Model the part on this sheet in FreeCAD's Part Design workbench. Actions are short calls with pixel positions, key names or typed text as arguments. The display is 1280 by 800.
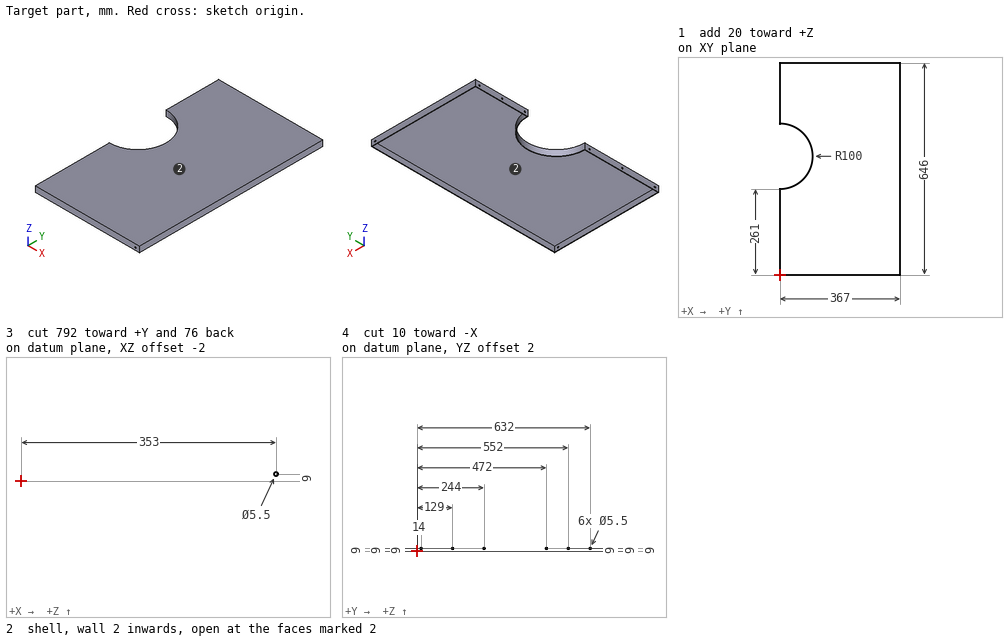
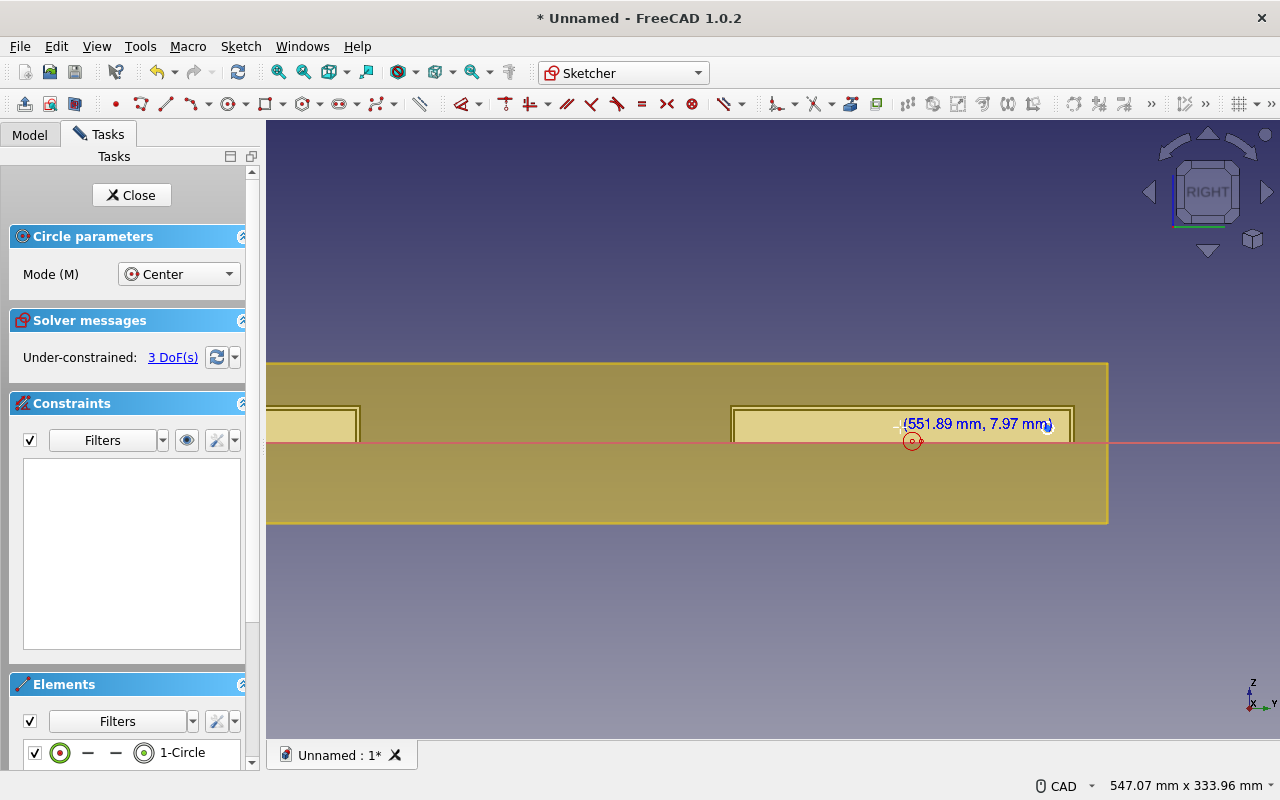
click(899, 427)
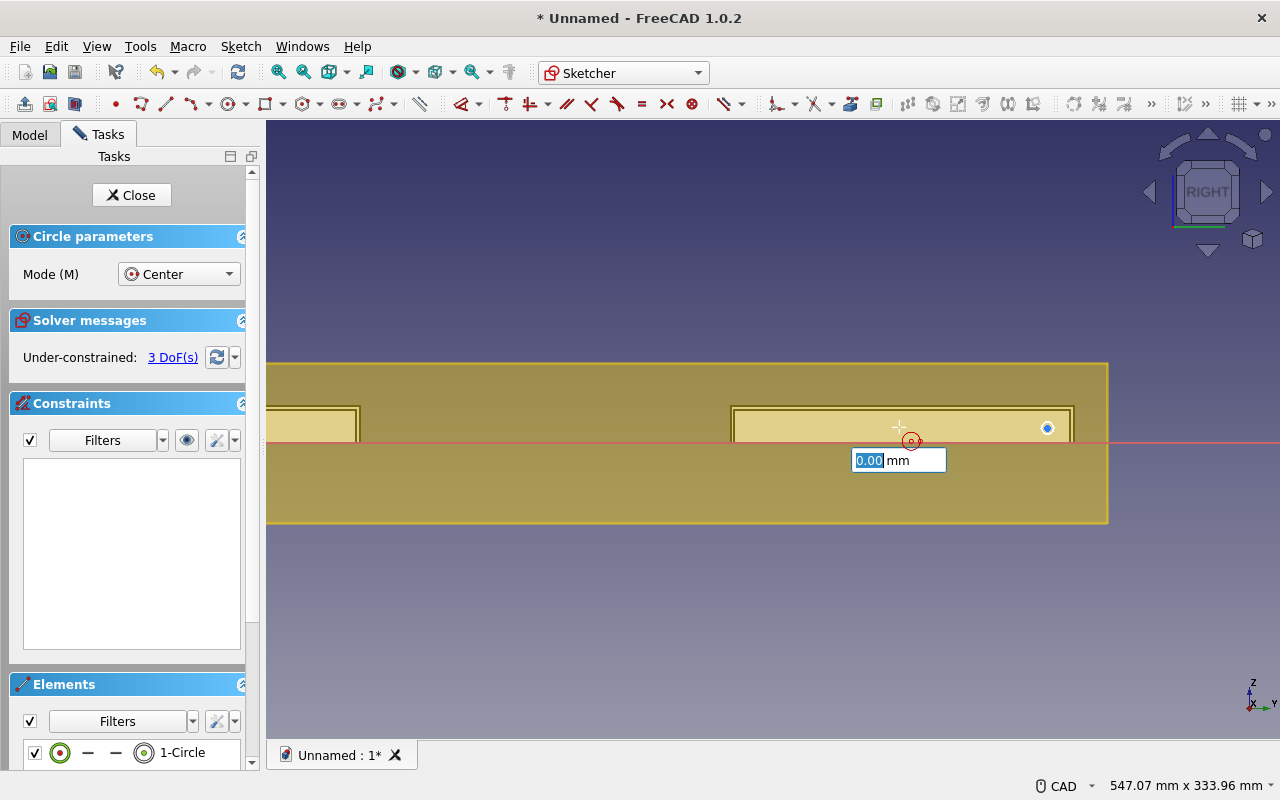
scroll(903, 423, up, 6)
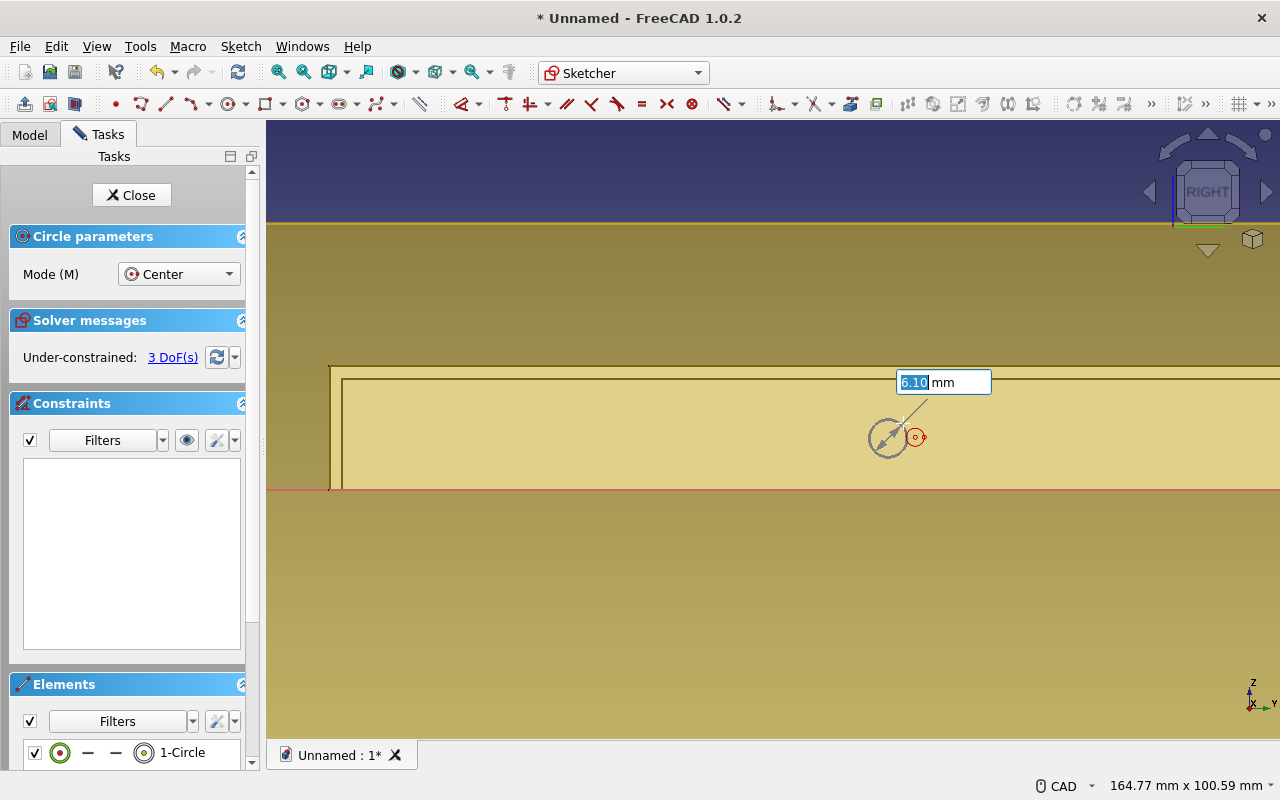
click(902, 422)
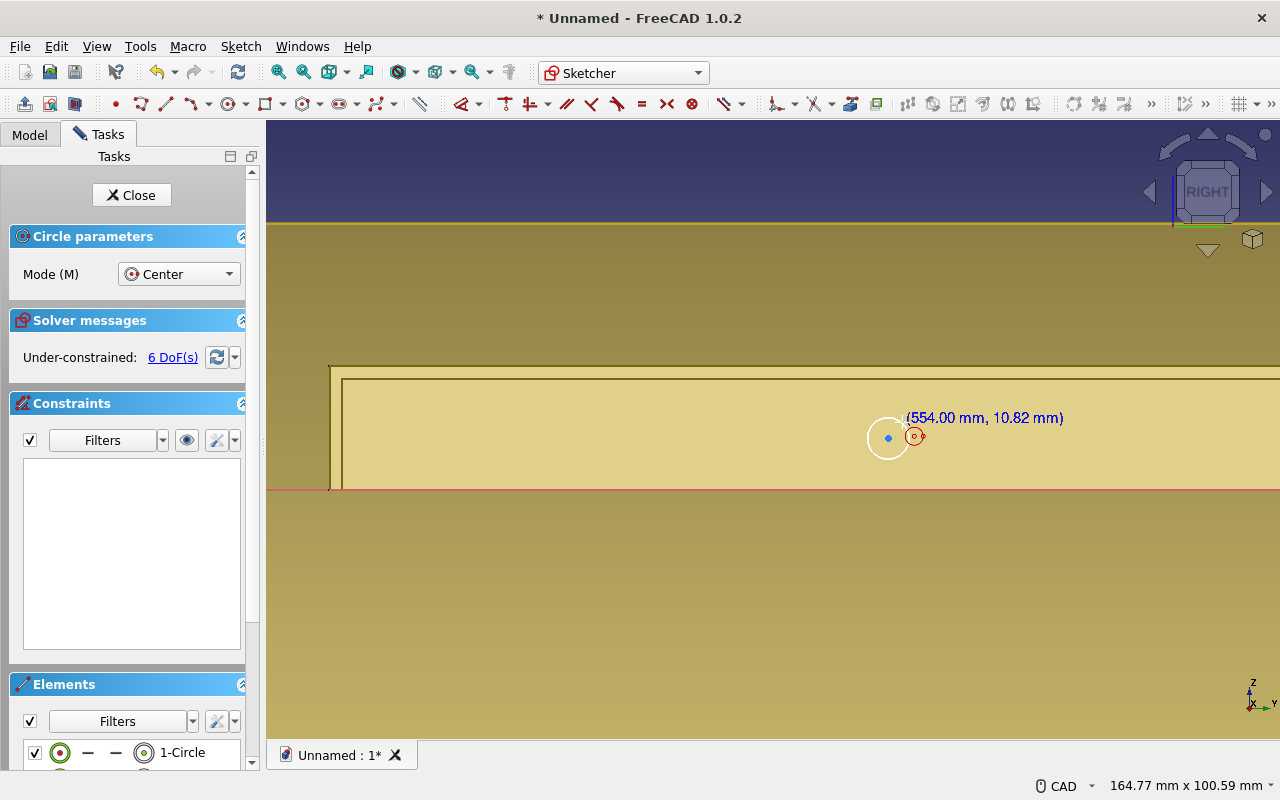
scroll(397, 434, up, 2)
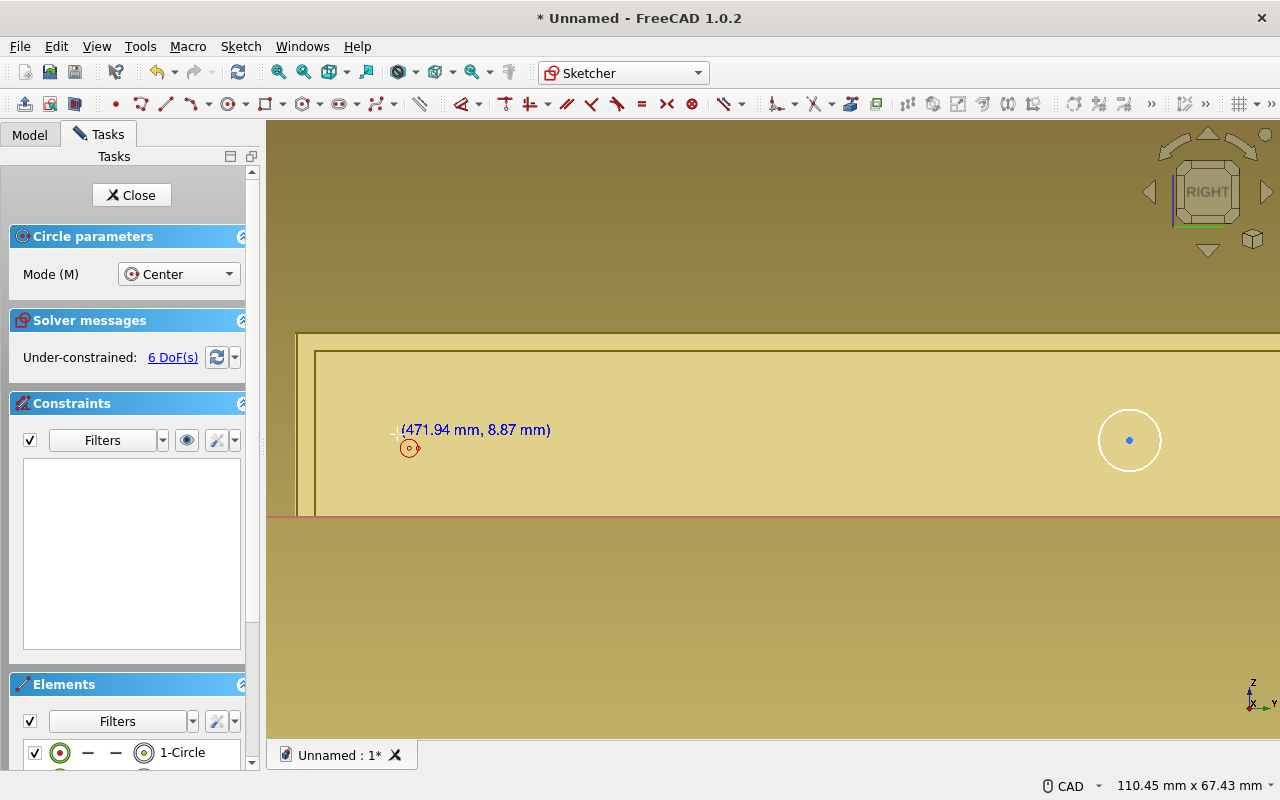
scroll(877, 426, down, 12)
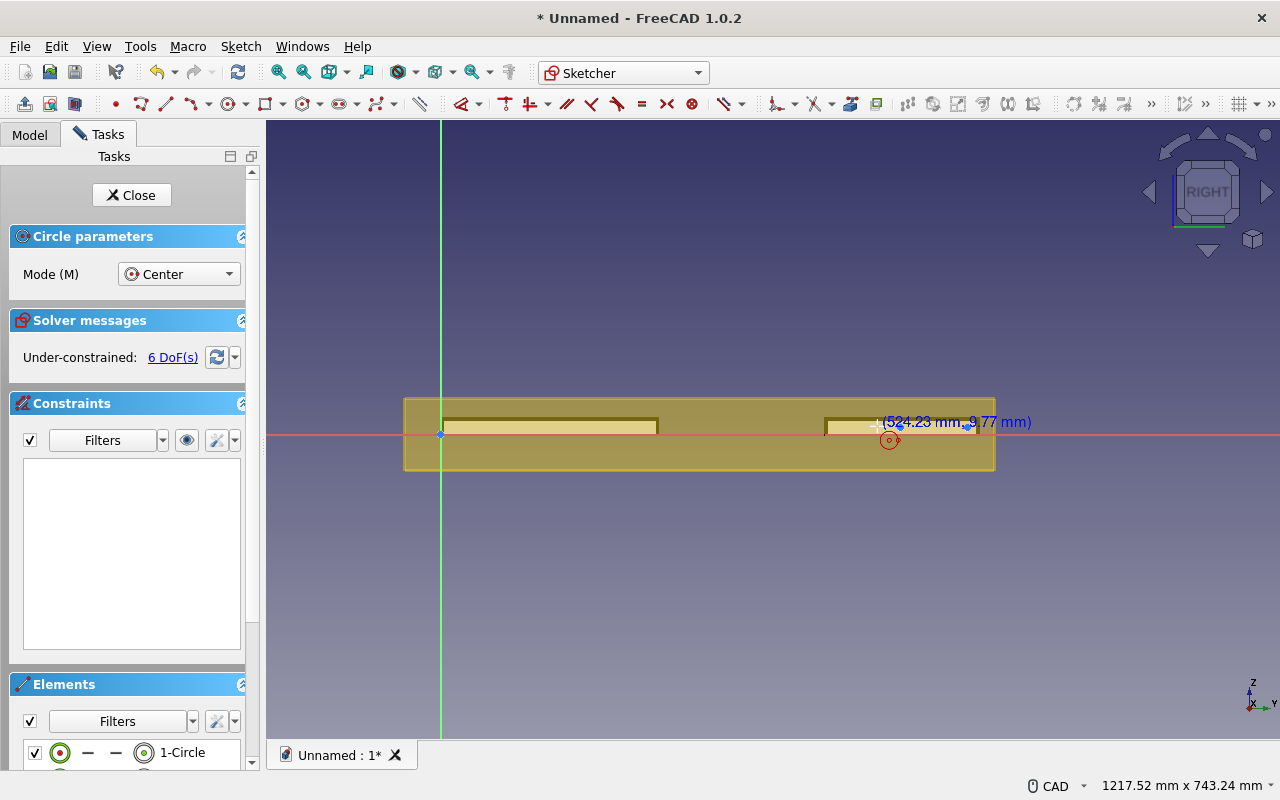
scroll(834, 427, up, 4)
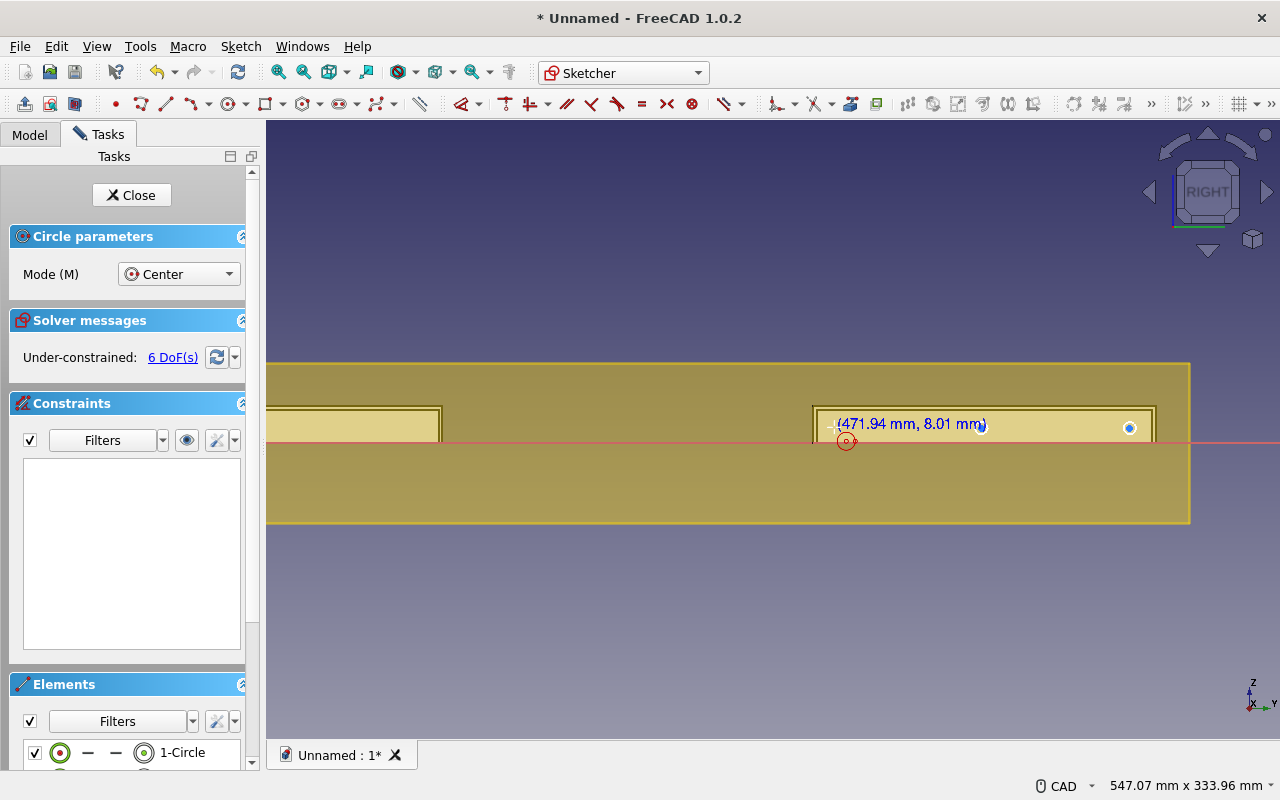
click(833, 427)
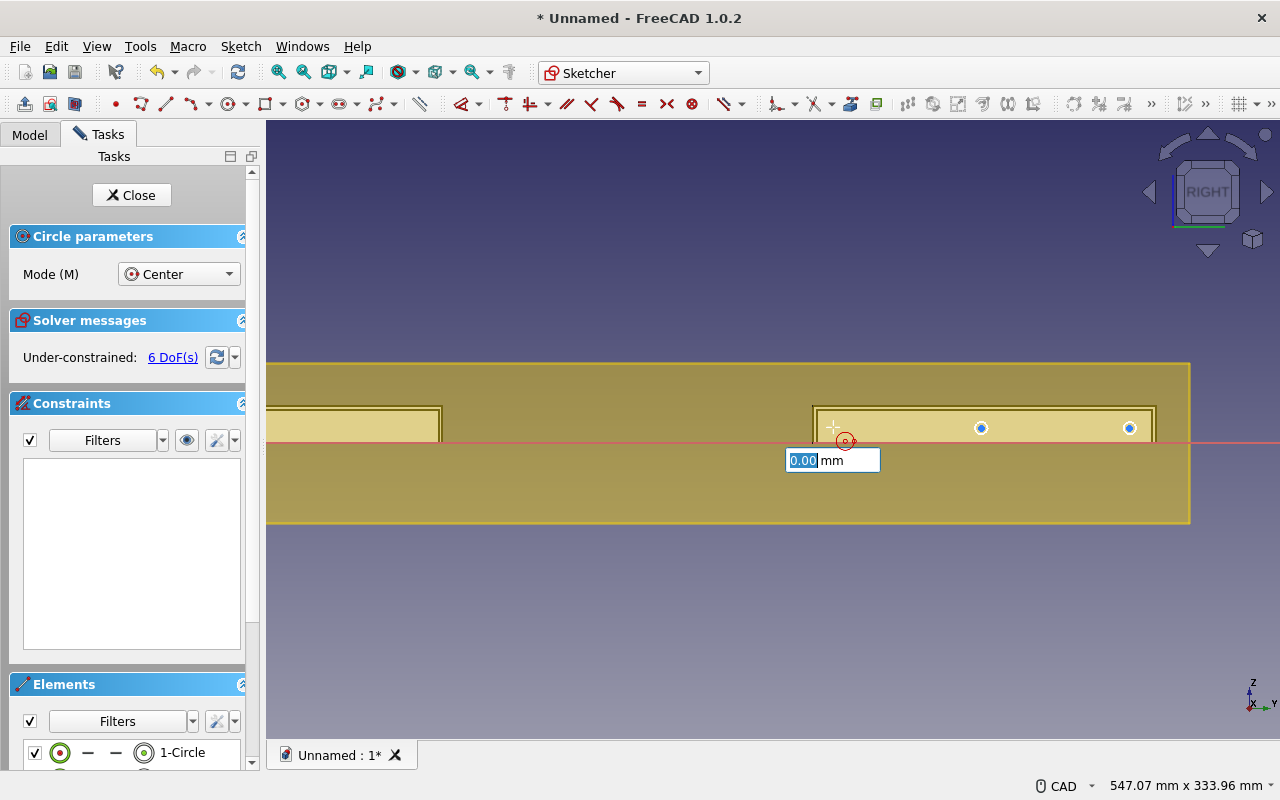
scroll(837, 423, up, 6)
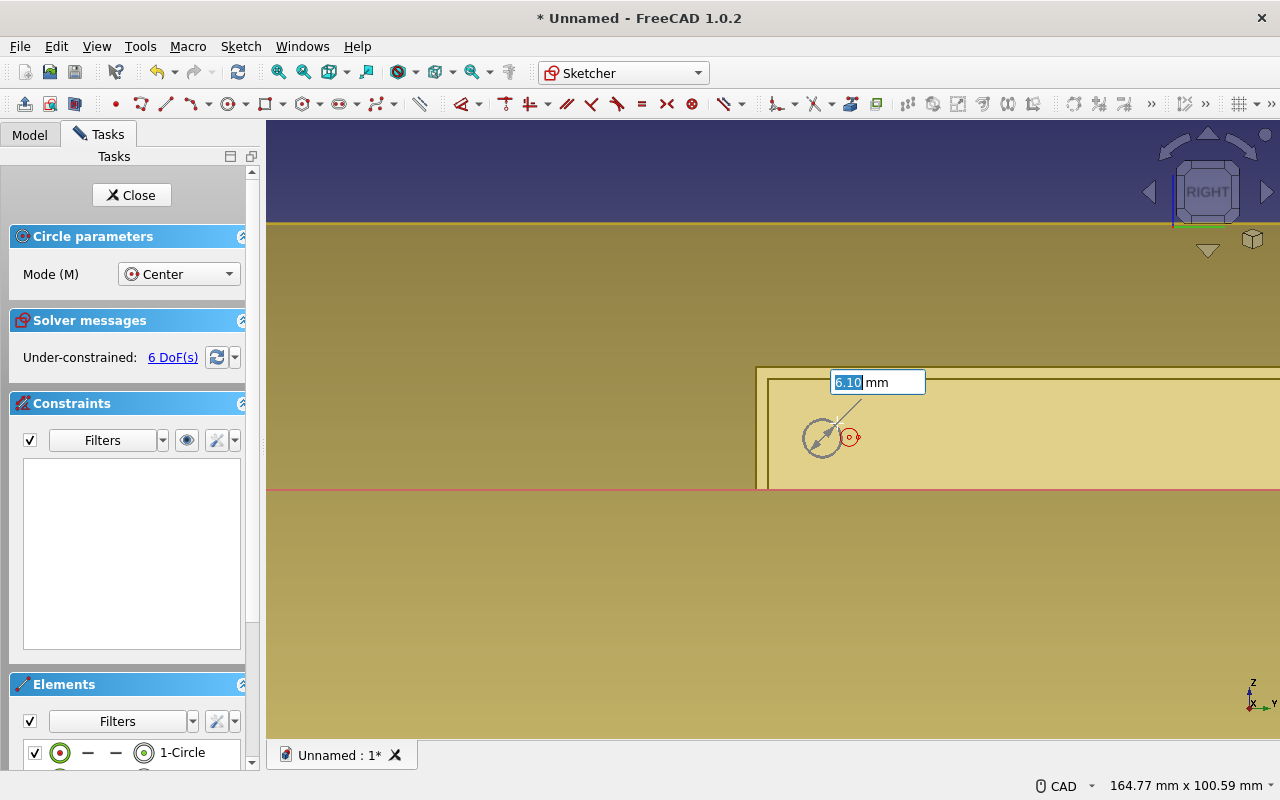
click(836, 422)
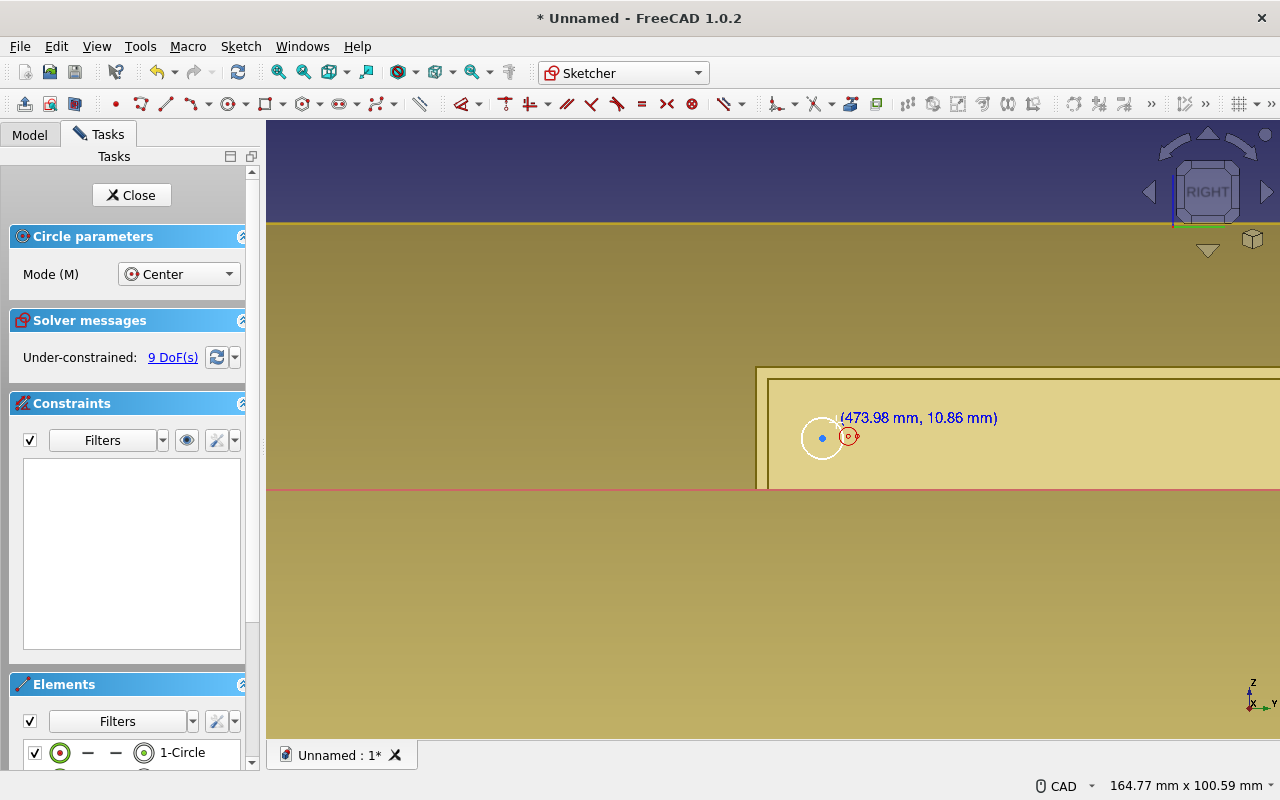
scroll(835, 426, down, 10)